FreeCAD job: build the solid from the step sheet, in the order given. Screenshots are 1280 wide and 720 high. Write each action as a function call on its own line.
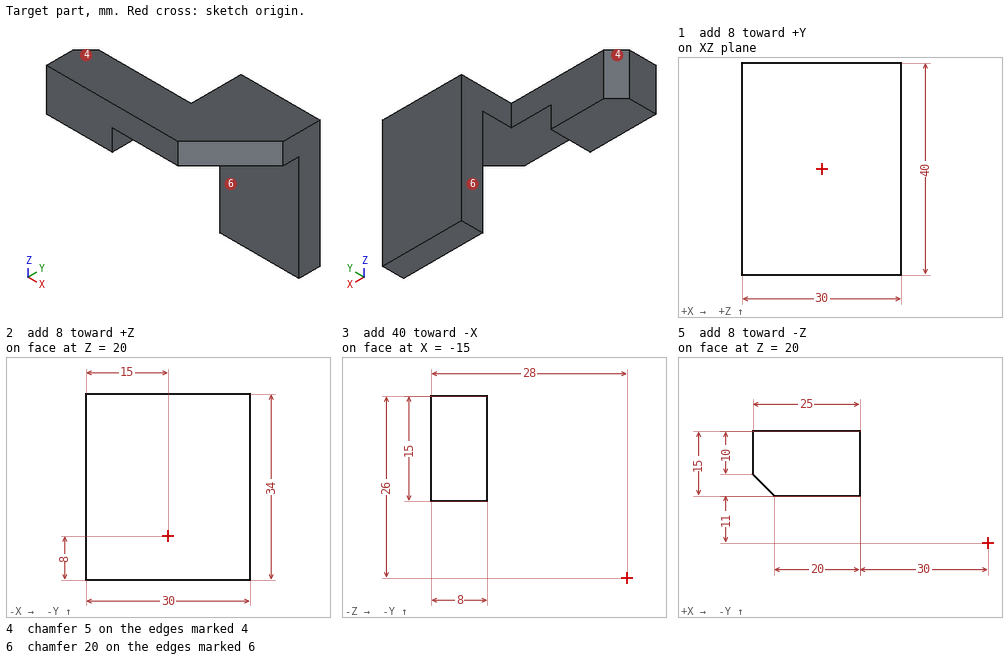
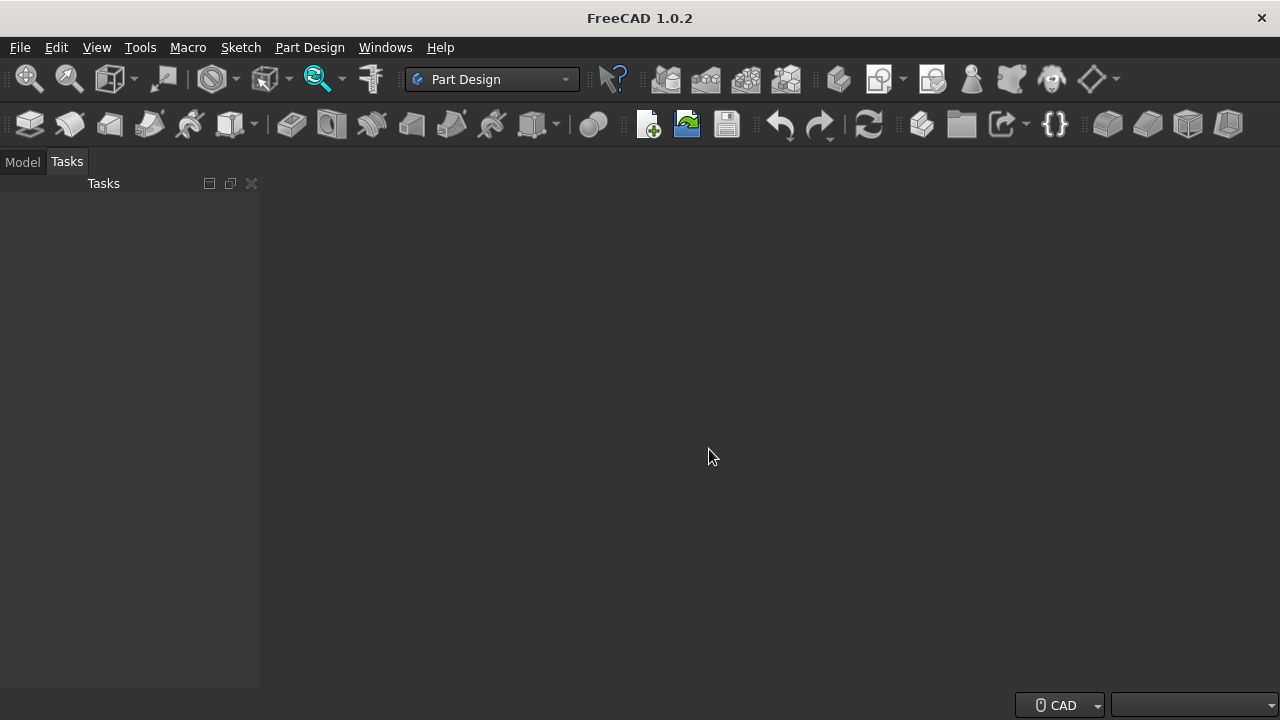
key(ctrl+n)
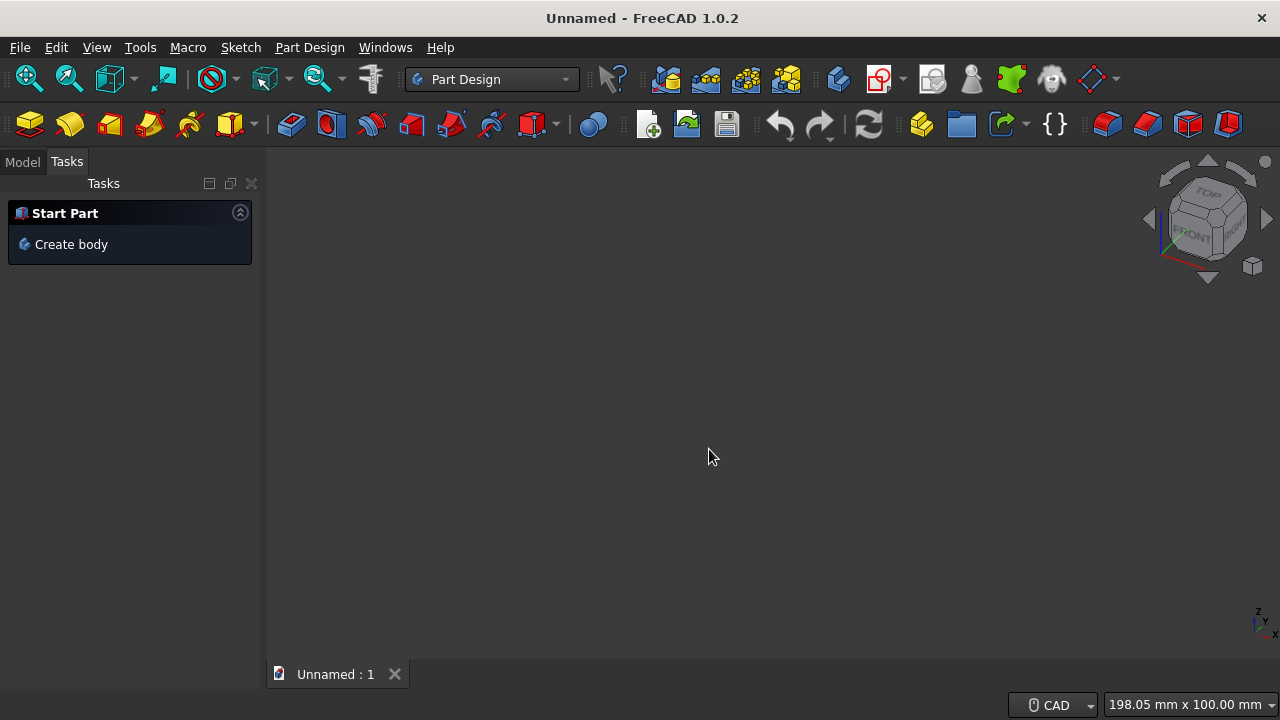
click(880, 80)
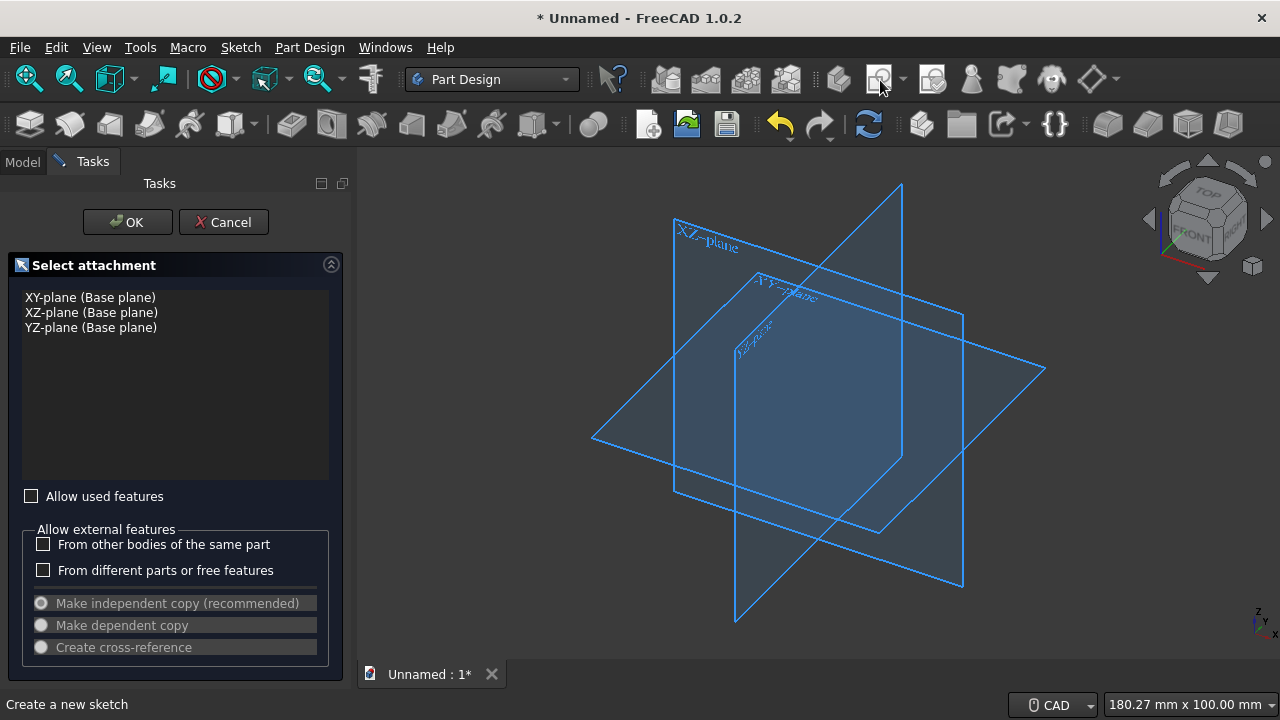
click(82, 312)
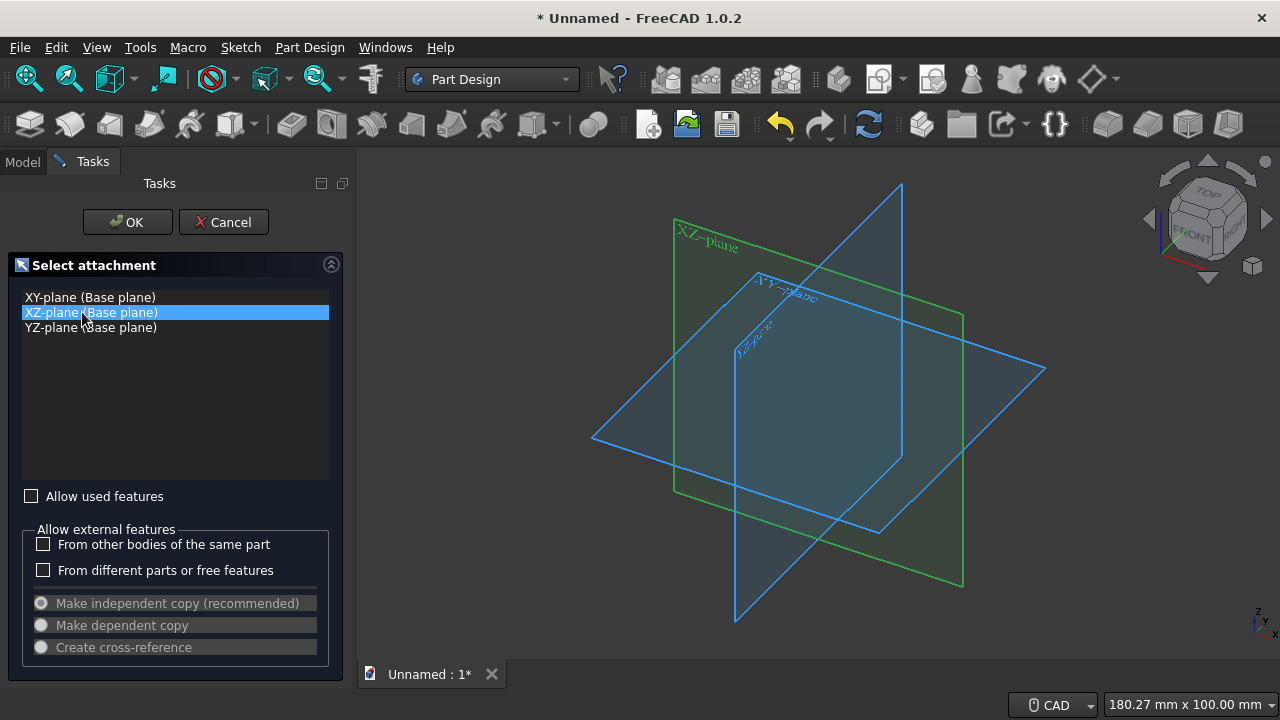
click(128, 222)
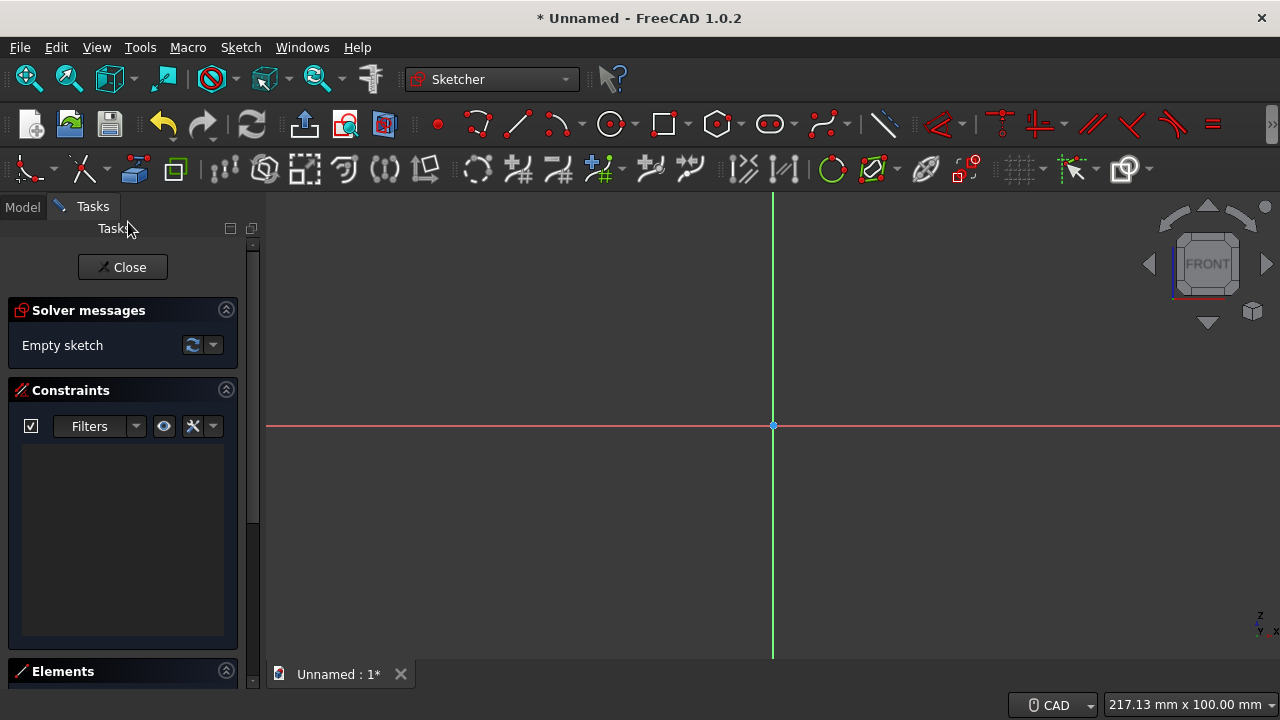
scroll(912, 425, up, 2)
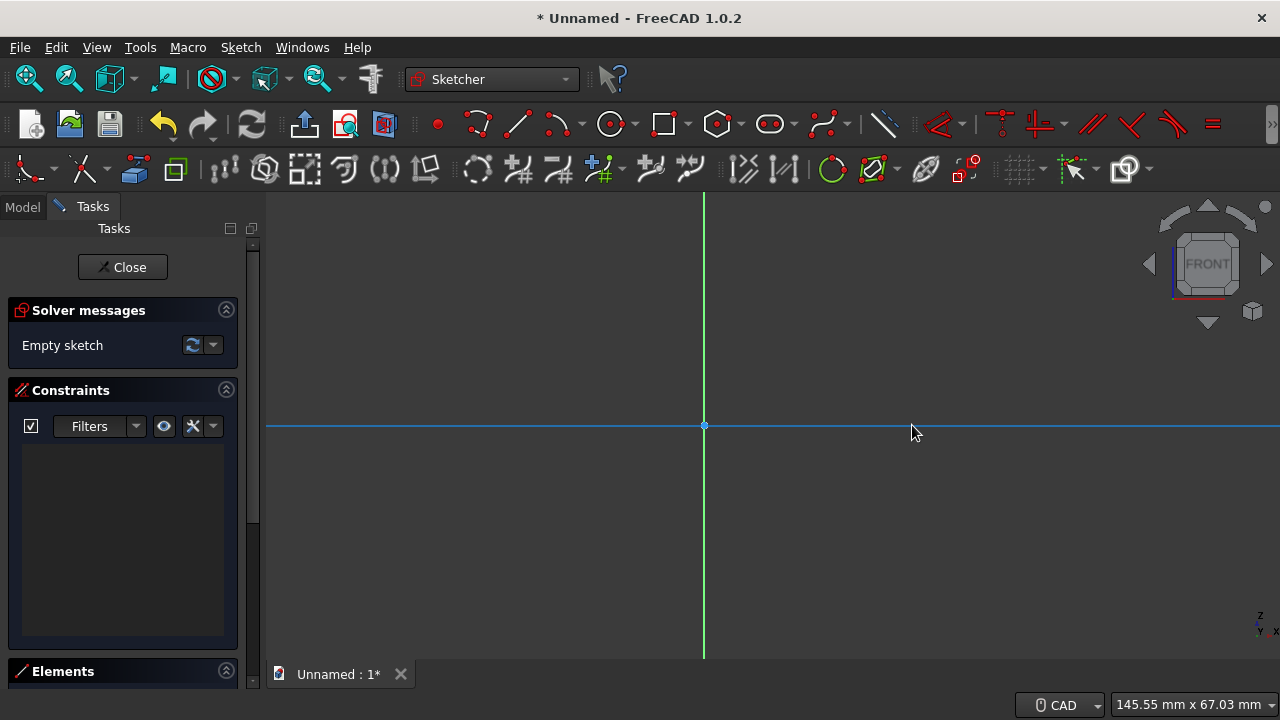
click(690, 124)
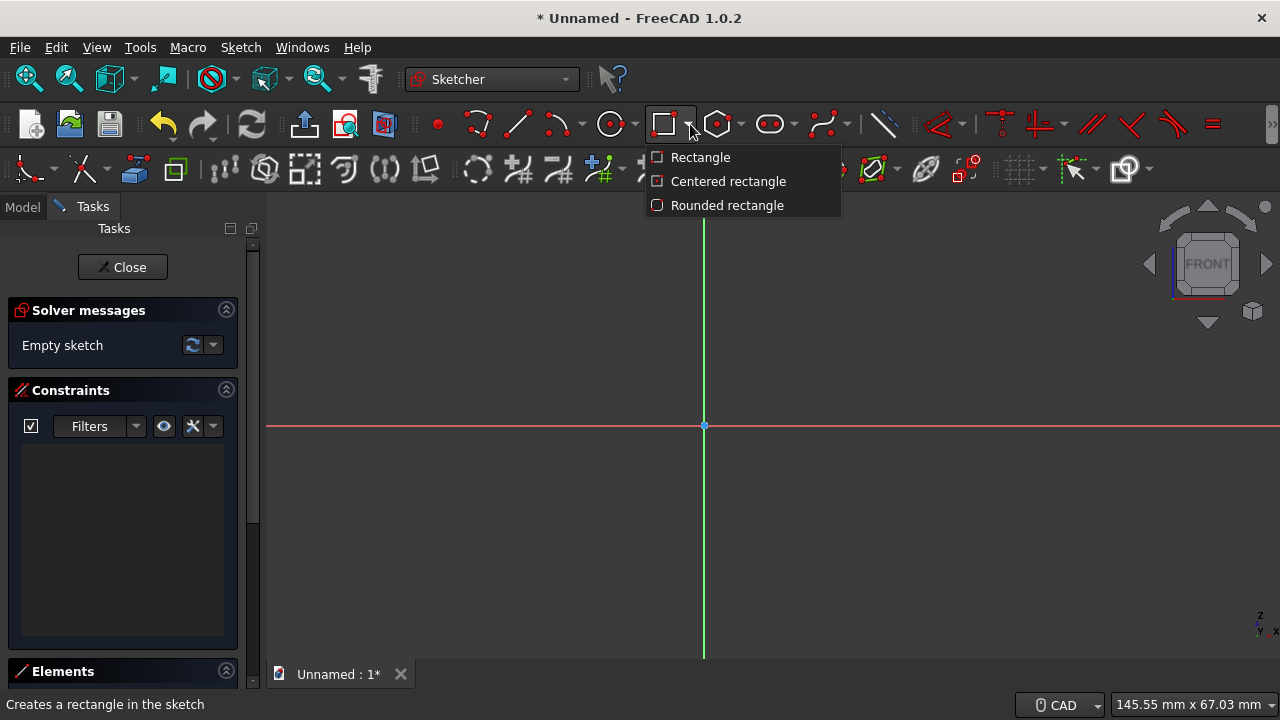
click(744, 181)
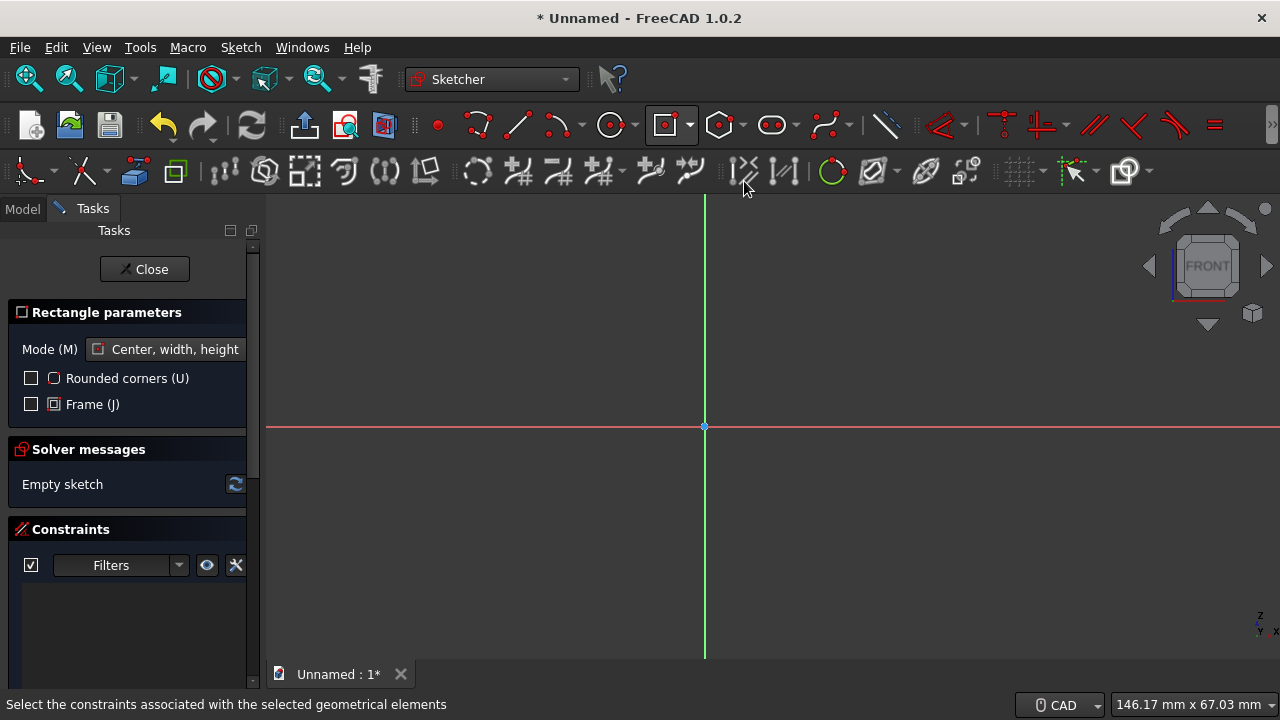
click(705, 426)
move(809, 288)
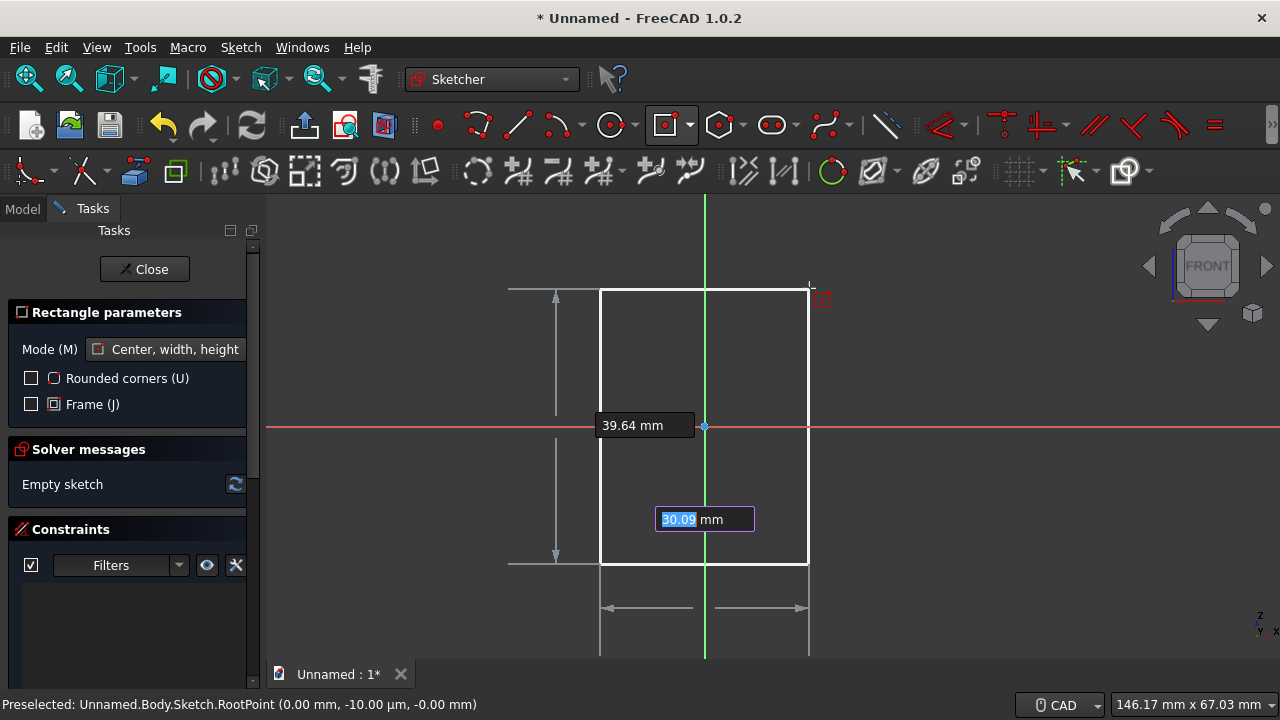
text(30)
key(Tab)
text(40)
key(Return)
key(Escape)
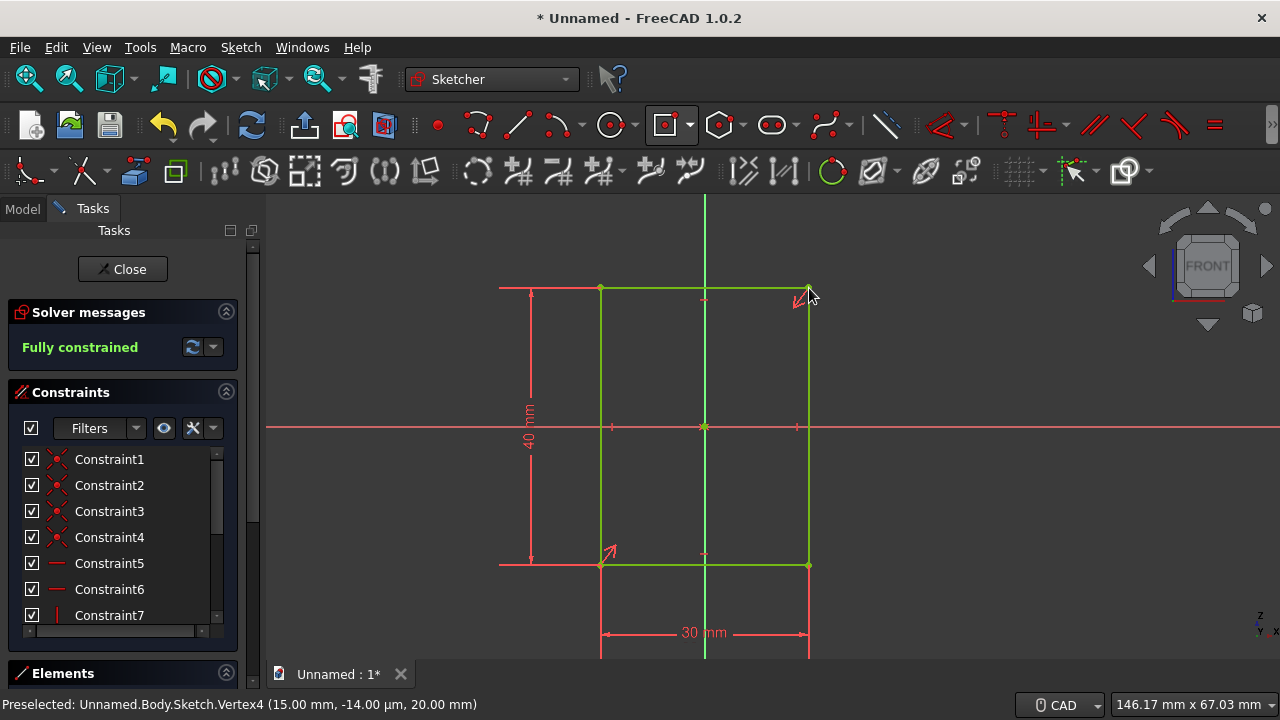
click(123, 269)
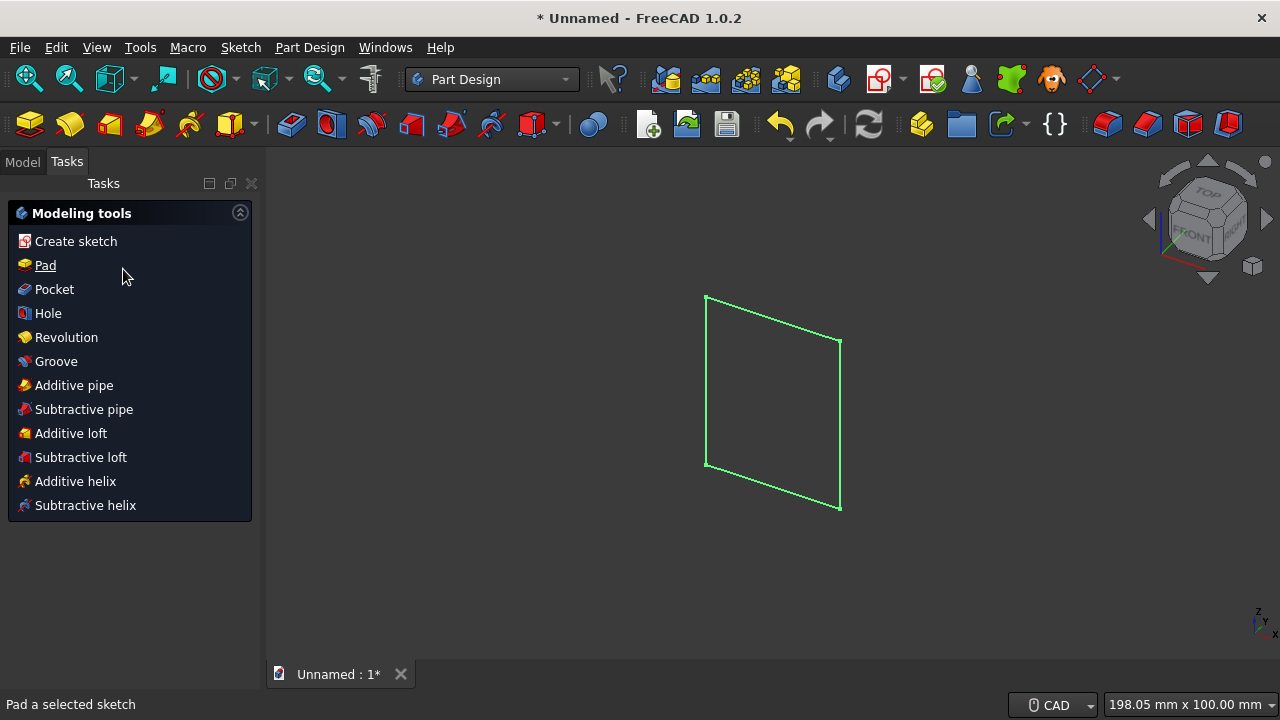
click(30, 124)